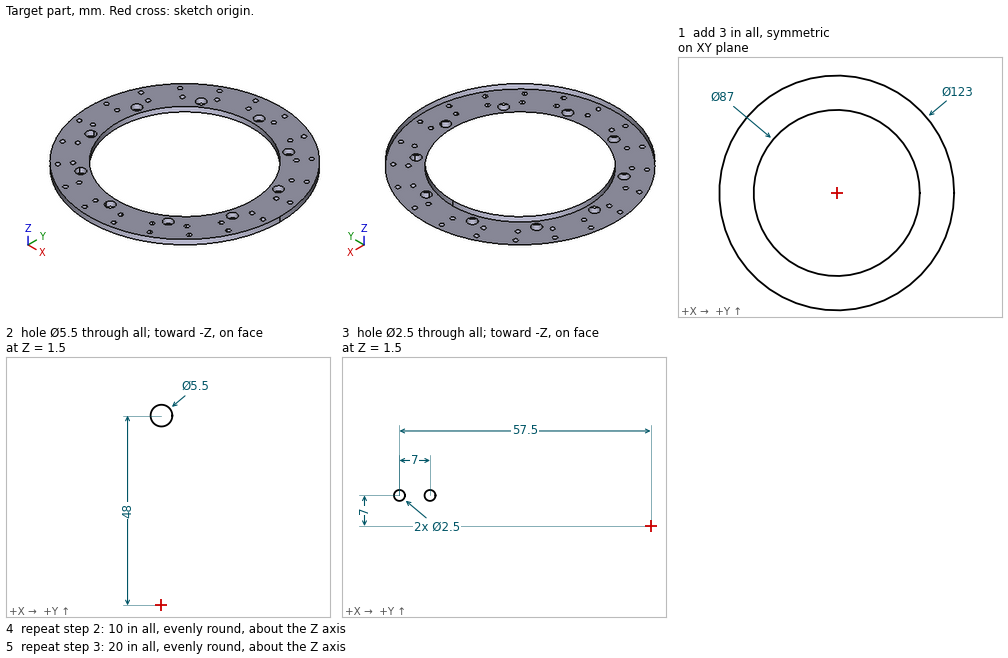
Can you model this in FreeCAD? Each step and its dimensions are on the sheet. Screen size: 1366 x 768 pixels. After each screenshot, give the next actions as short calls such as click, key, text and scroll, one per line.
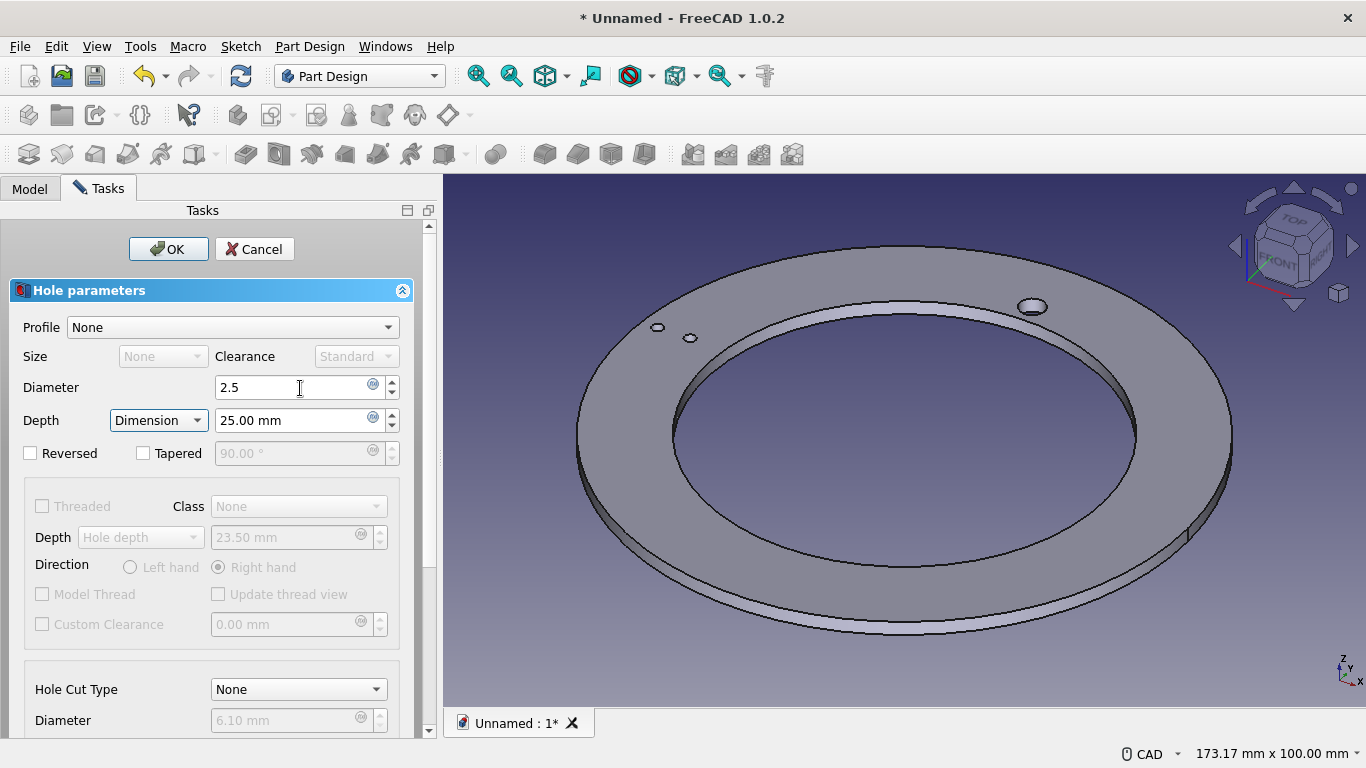
click(160, 420)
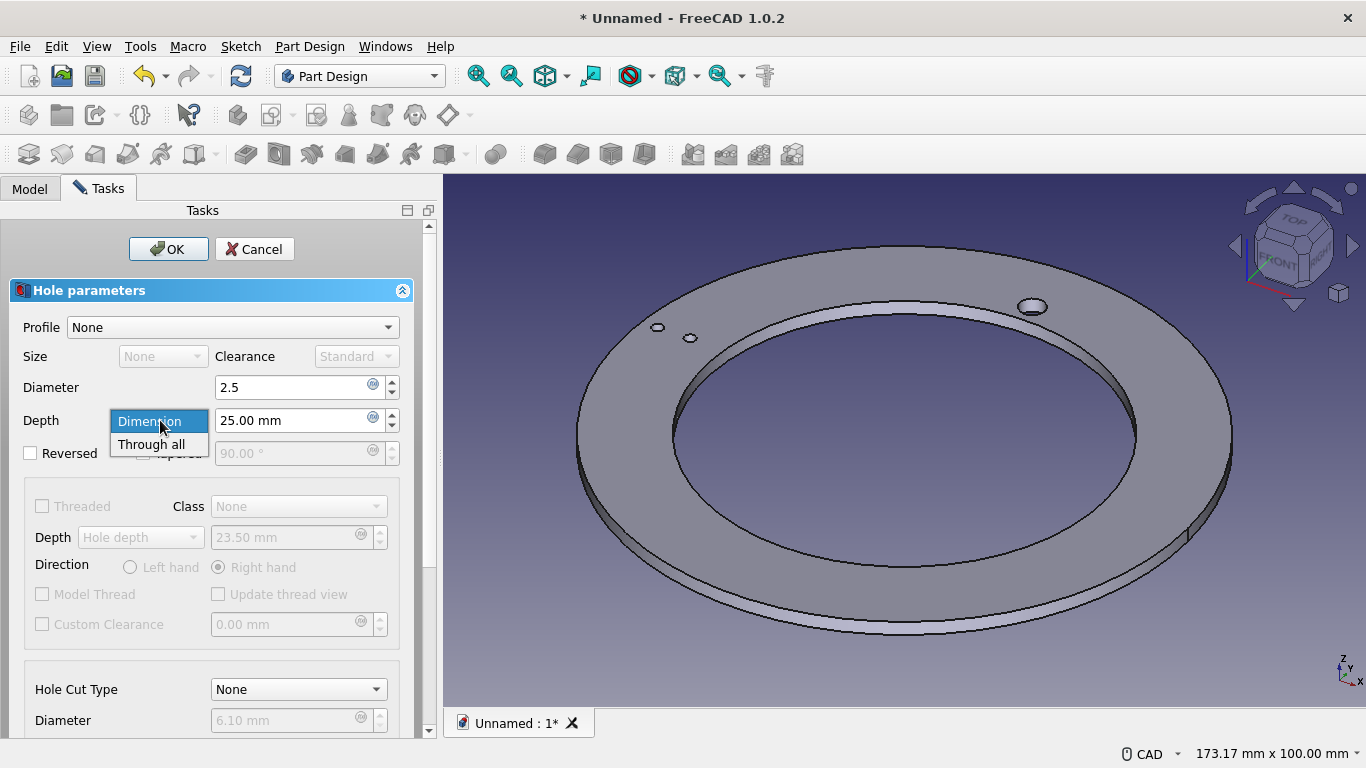
click(158, 444)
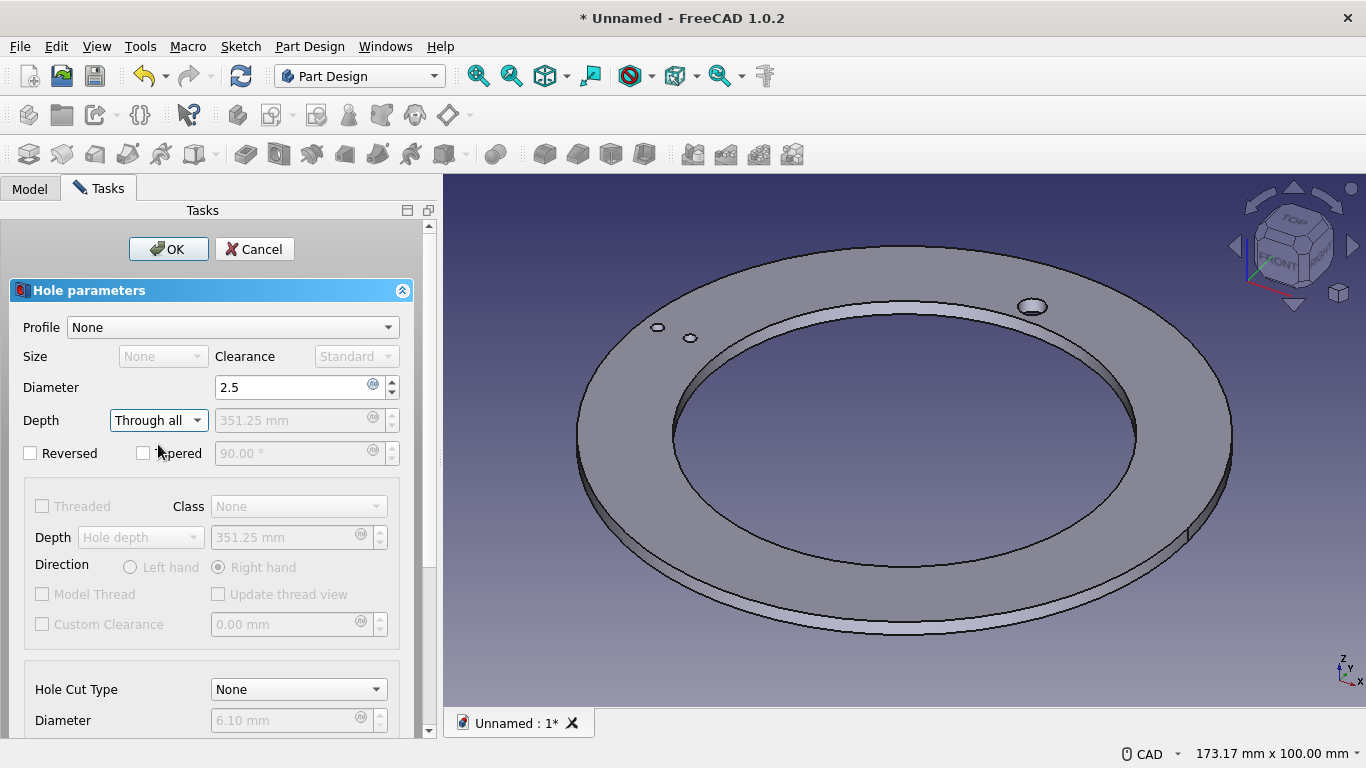
click(169, 249)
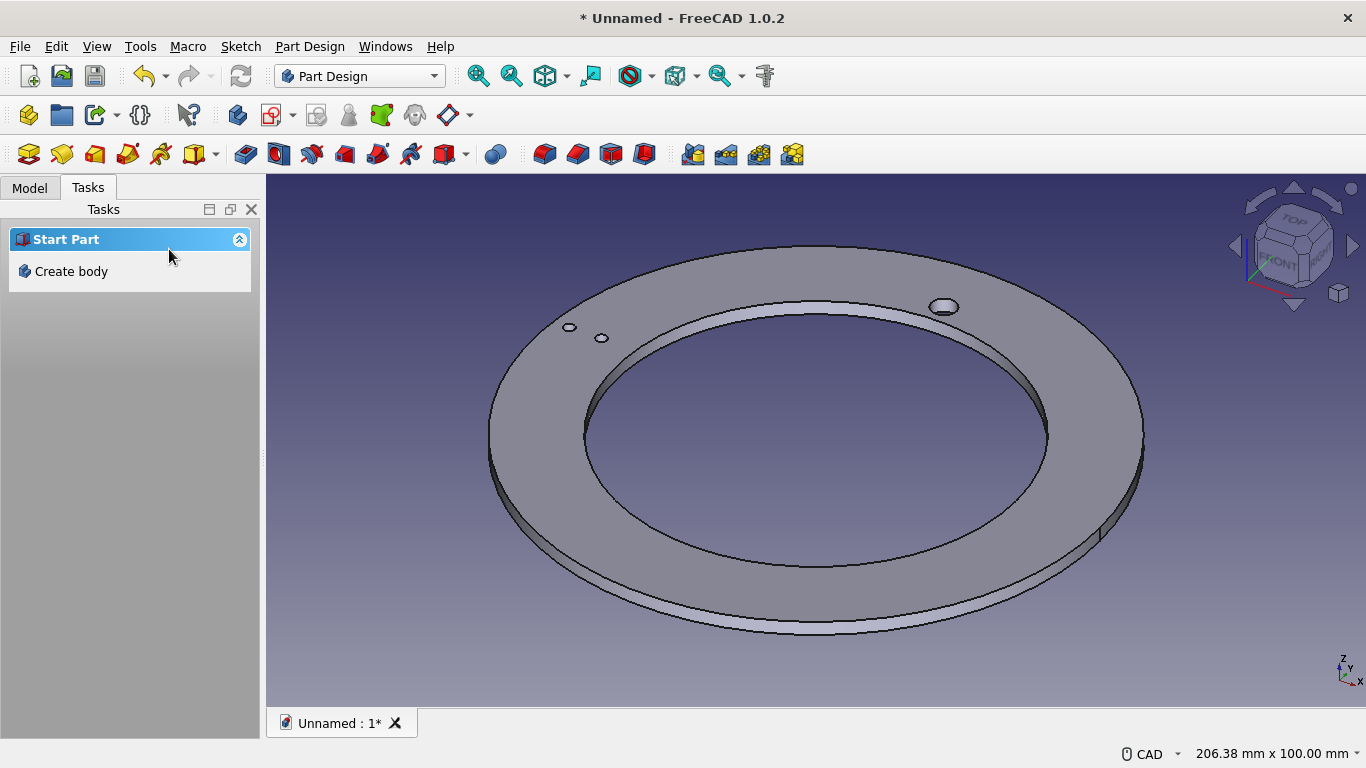
click(30, 188)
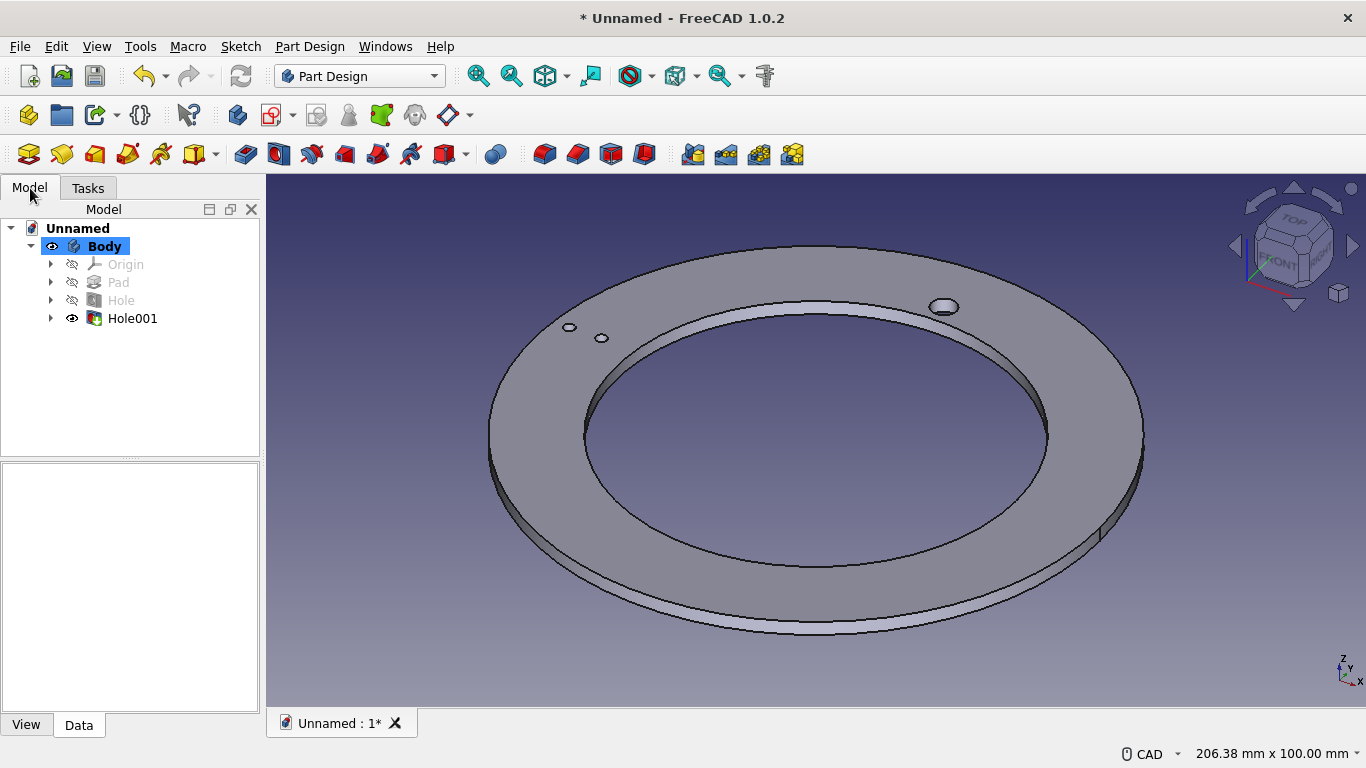
click(117, 300)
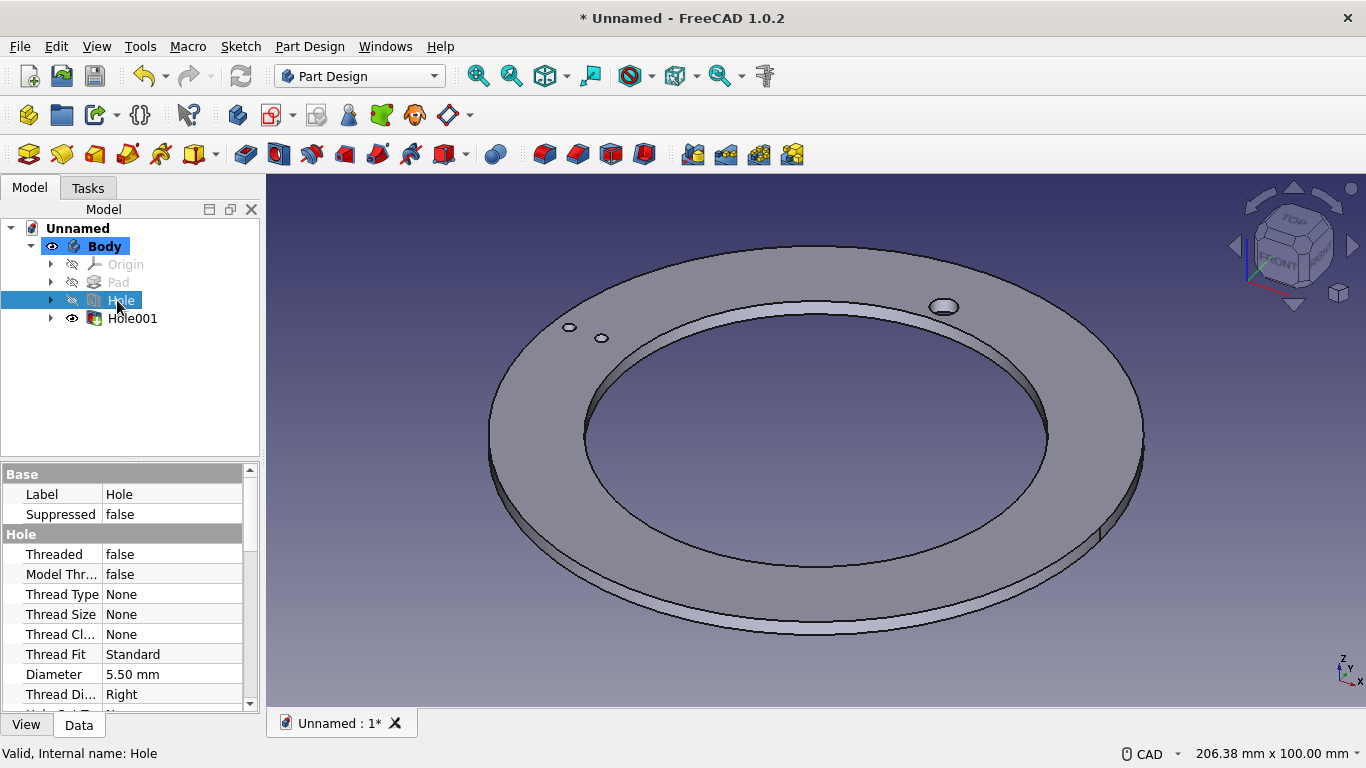
click(759, 154)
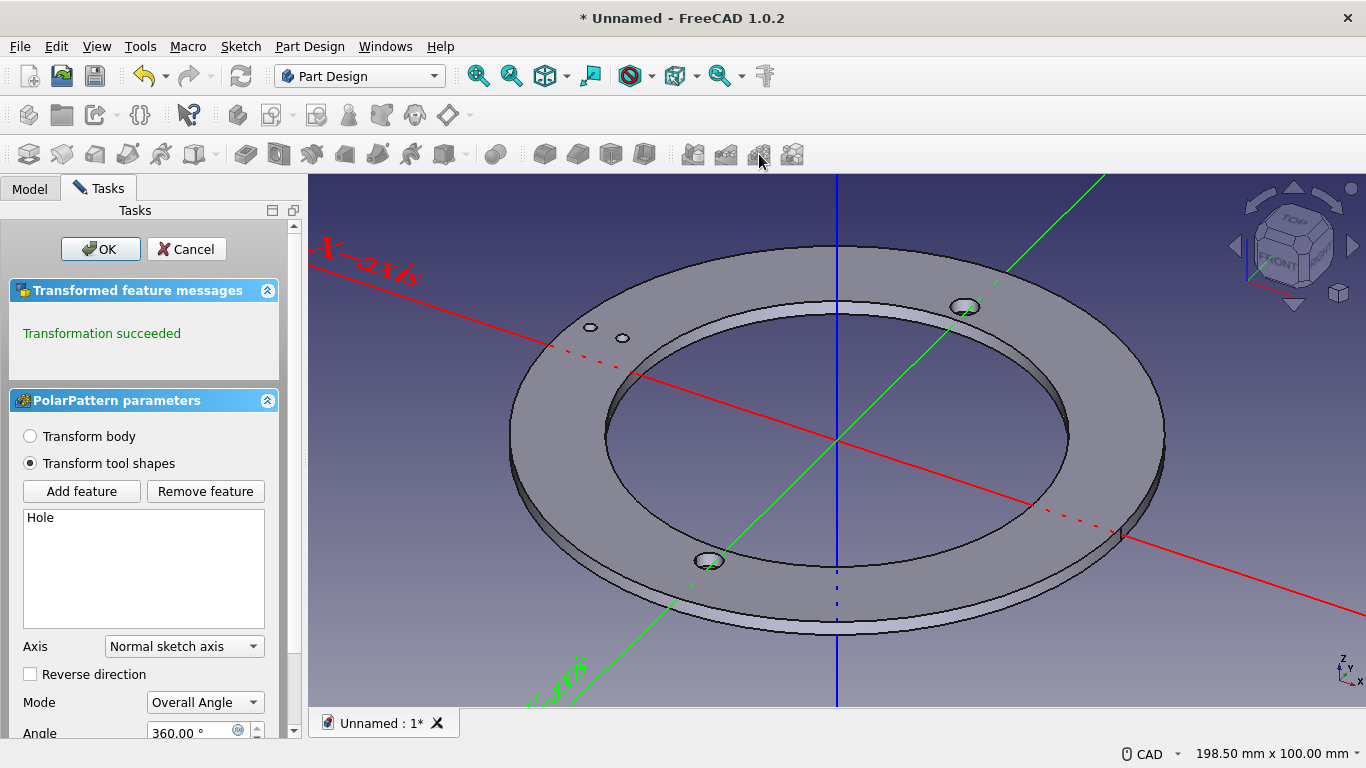
click(185, 646)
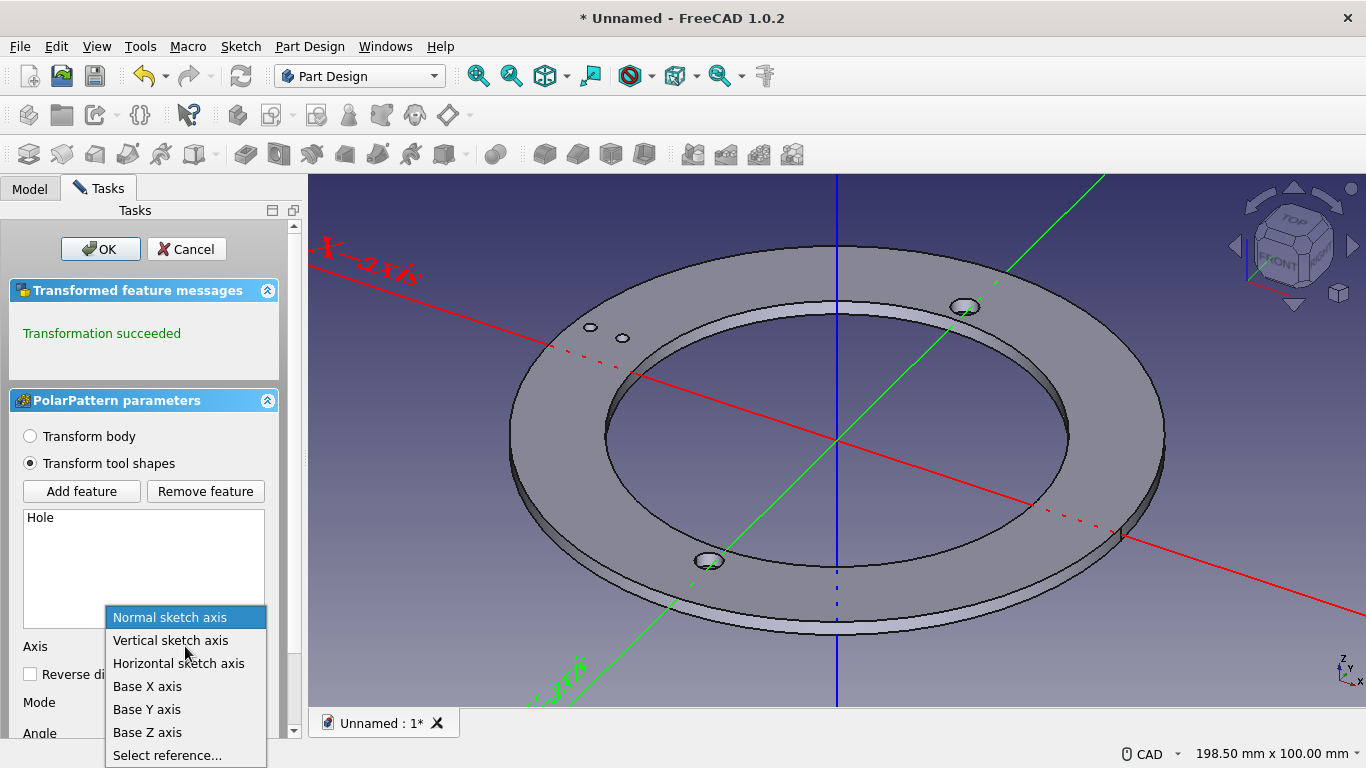
click(184, 732)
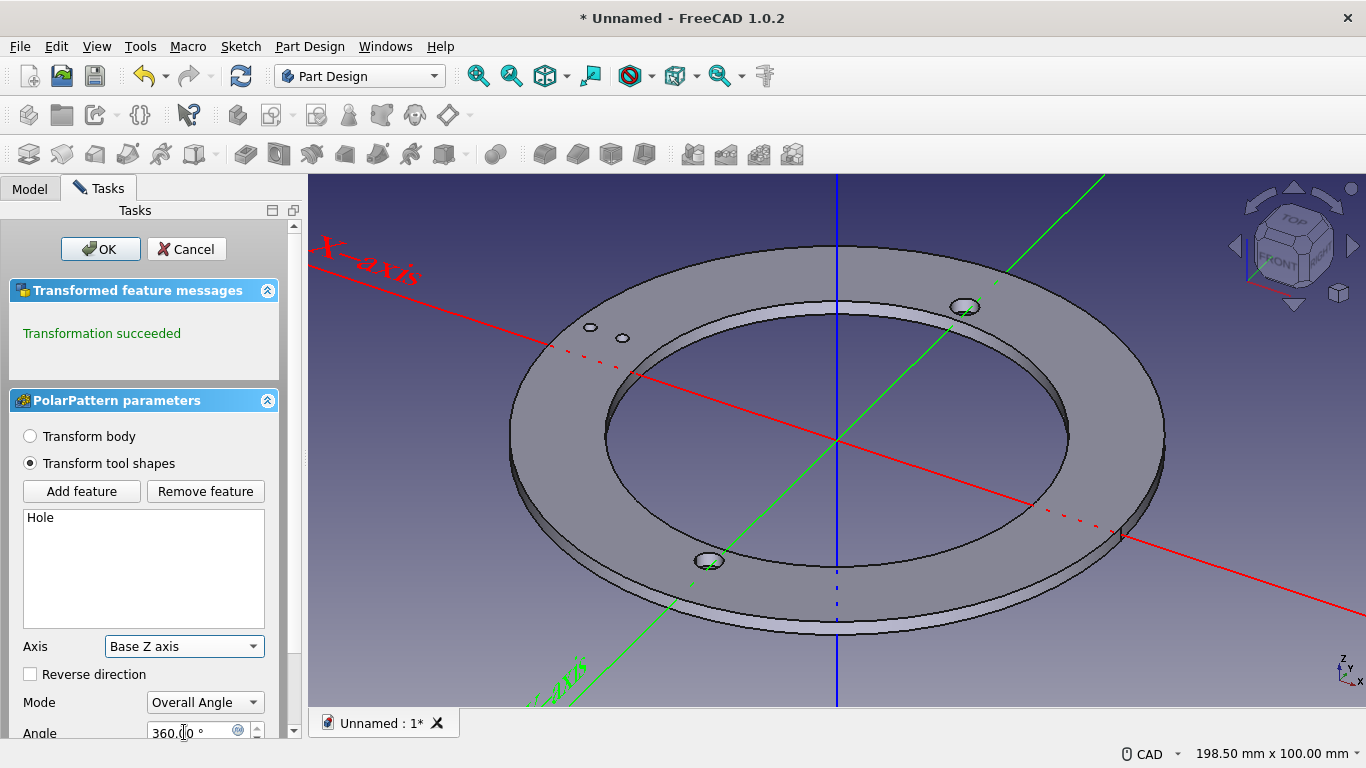
scroll(294, 479, down, 2)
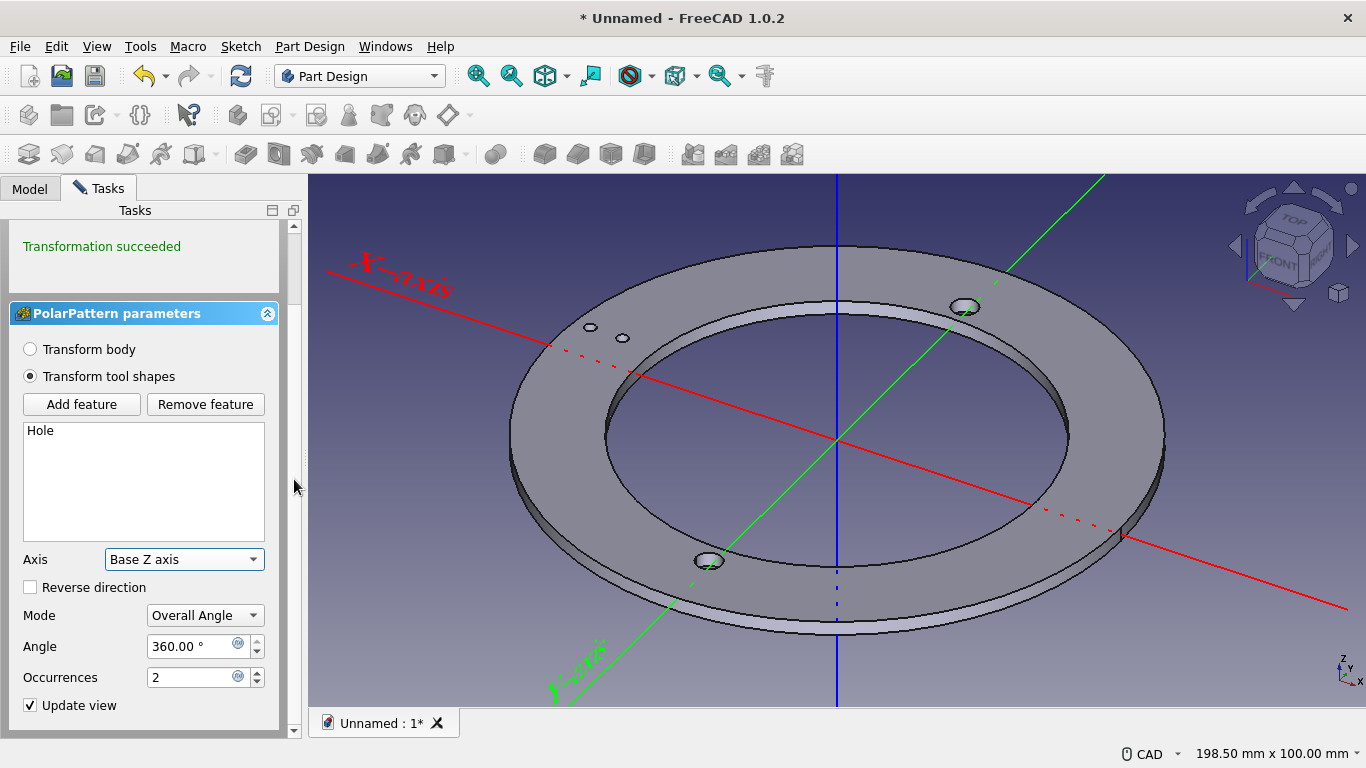
triple_click(199, 678)